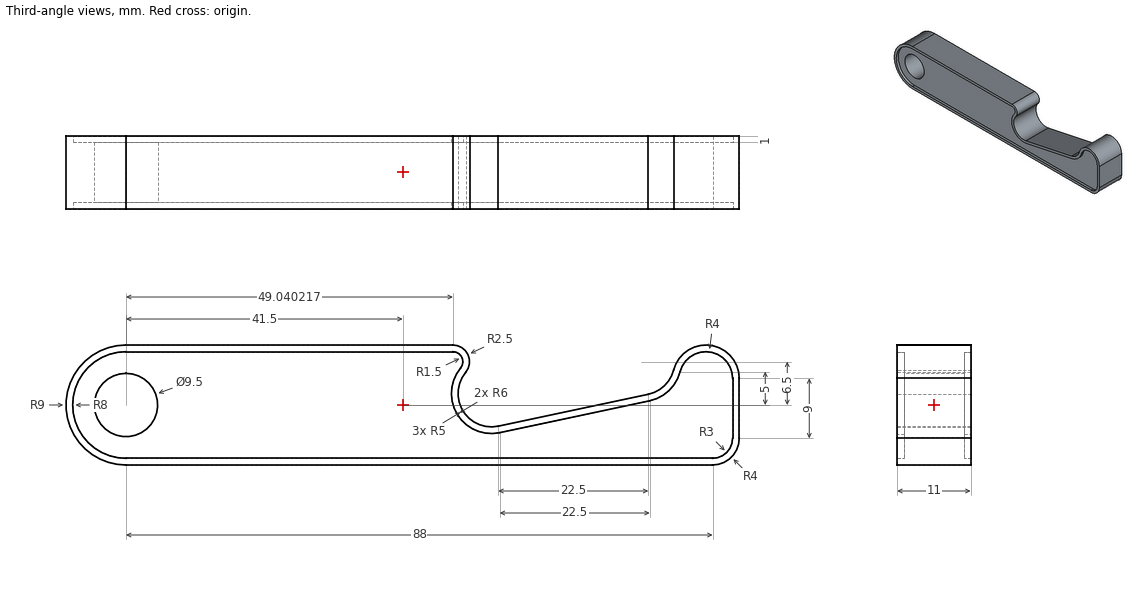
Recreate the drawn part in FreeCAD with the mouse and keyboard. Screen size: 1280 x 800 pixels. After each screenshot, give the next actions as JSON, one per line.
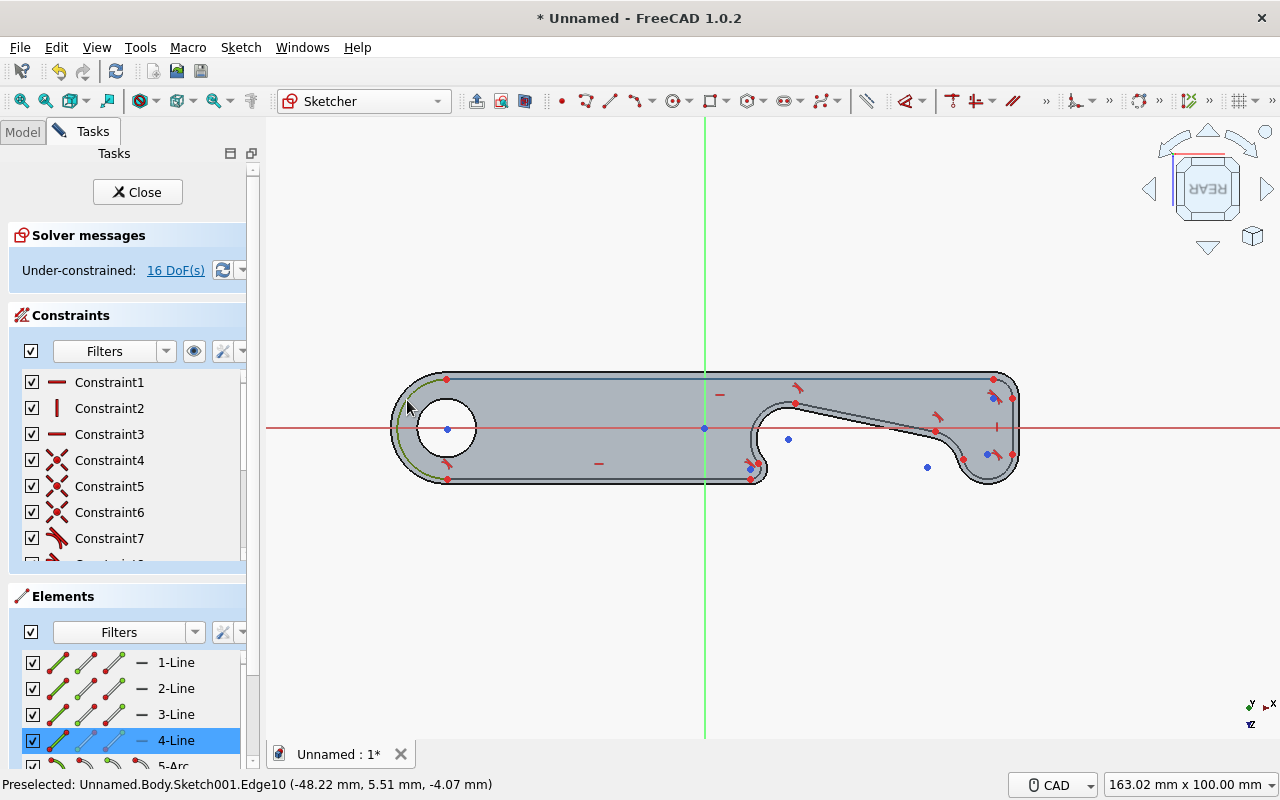
{"action": "key", "text": "t"}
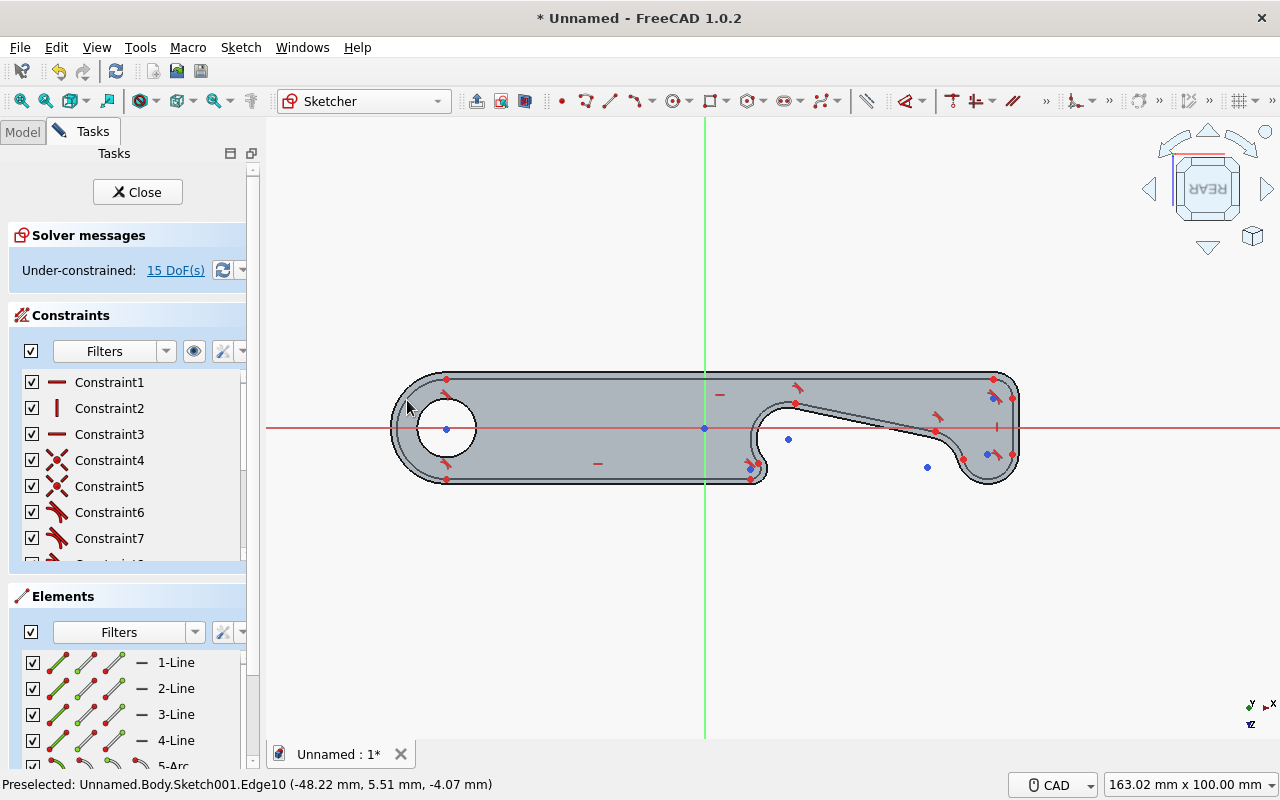
{"action": "scroll", "coordinate": [760, 474], "scroll_direction": "up", "scroll_amount": 2}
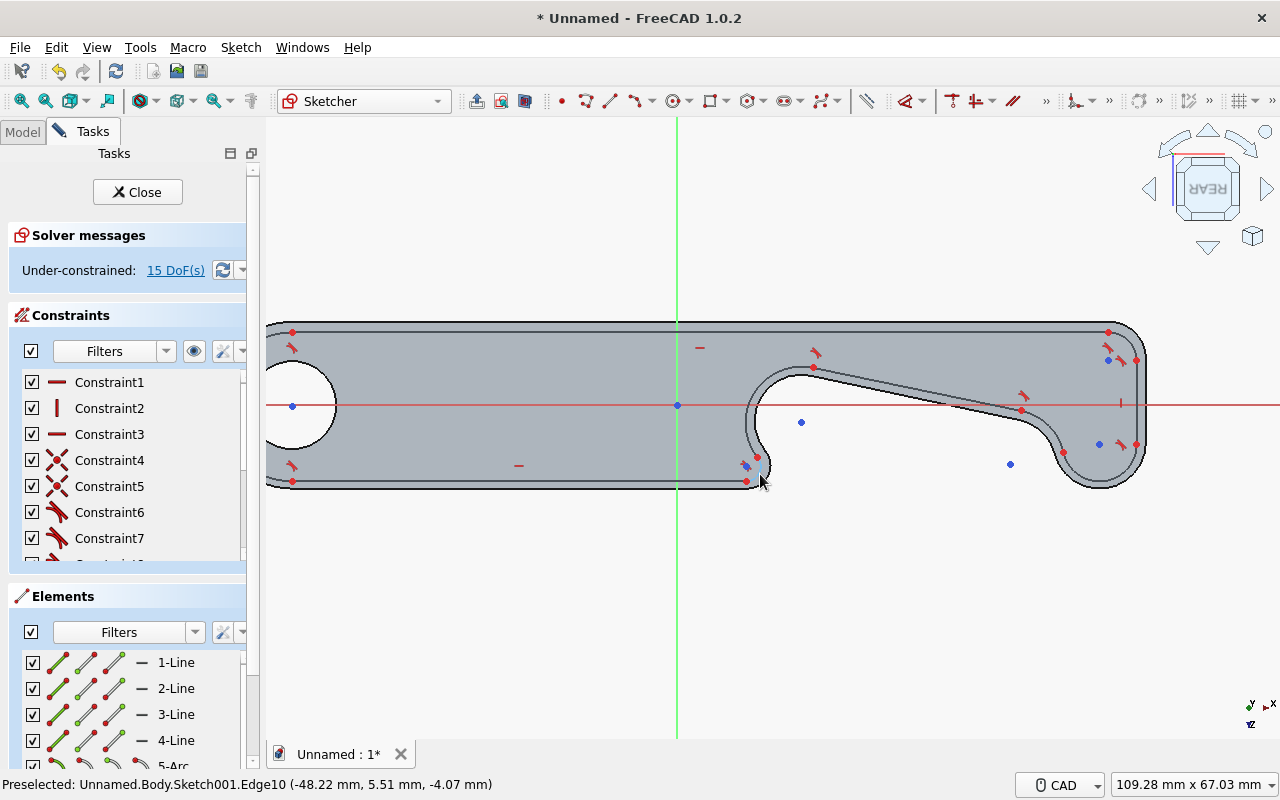
{"action": "left_click", "coordinate": [759, 473]}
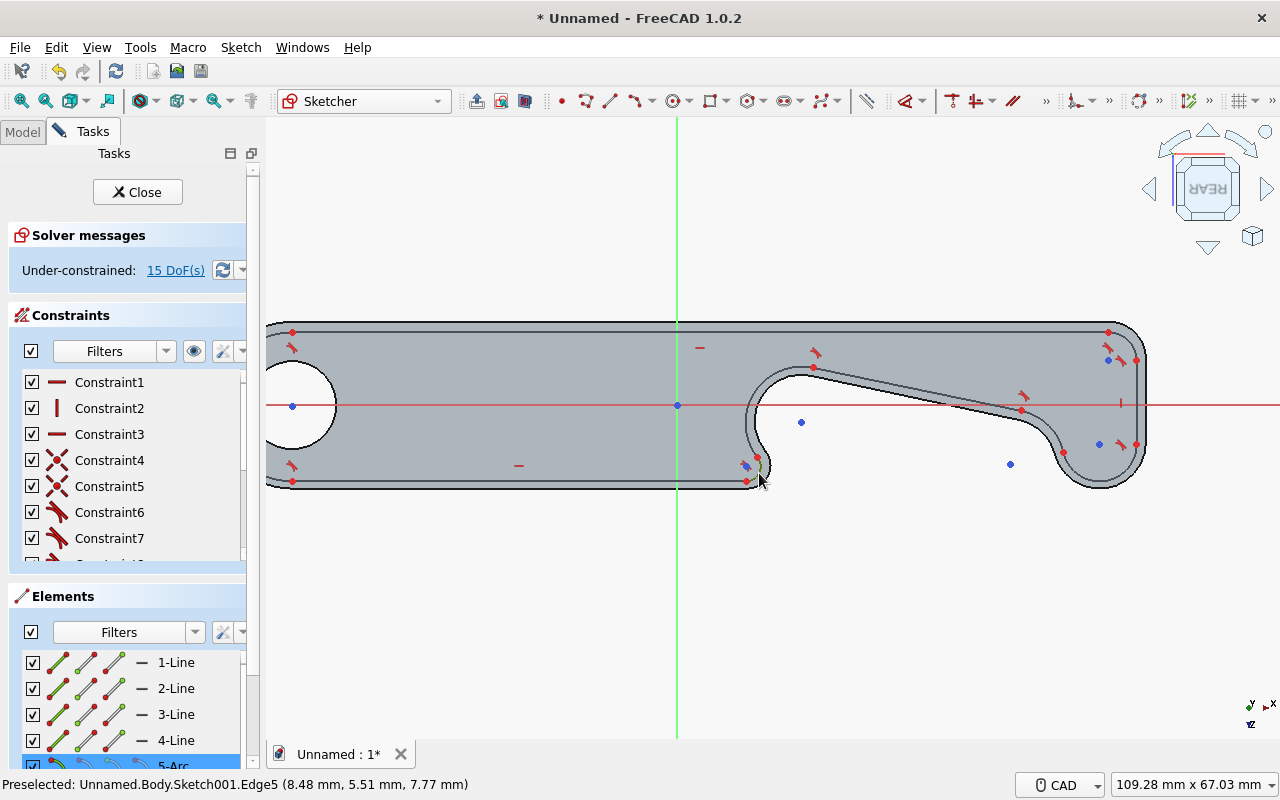
{"action": "left_click", "coordinate": [773, 374]}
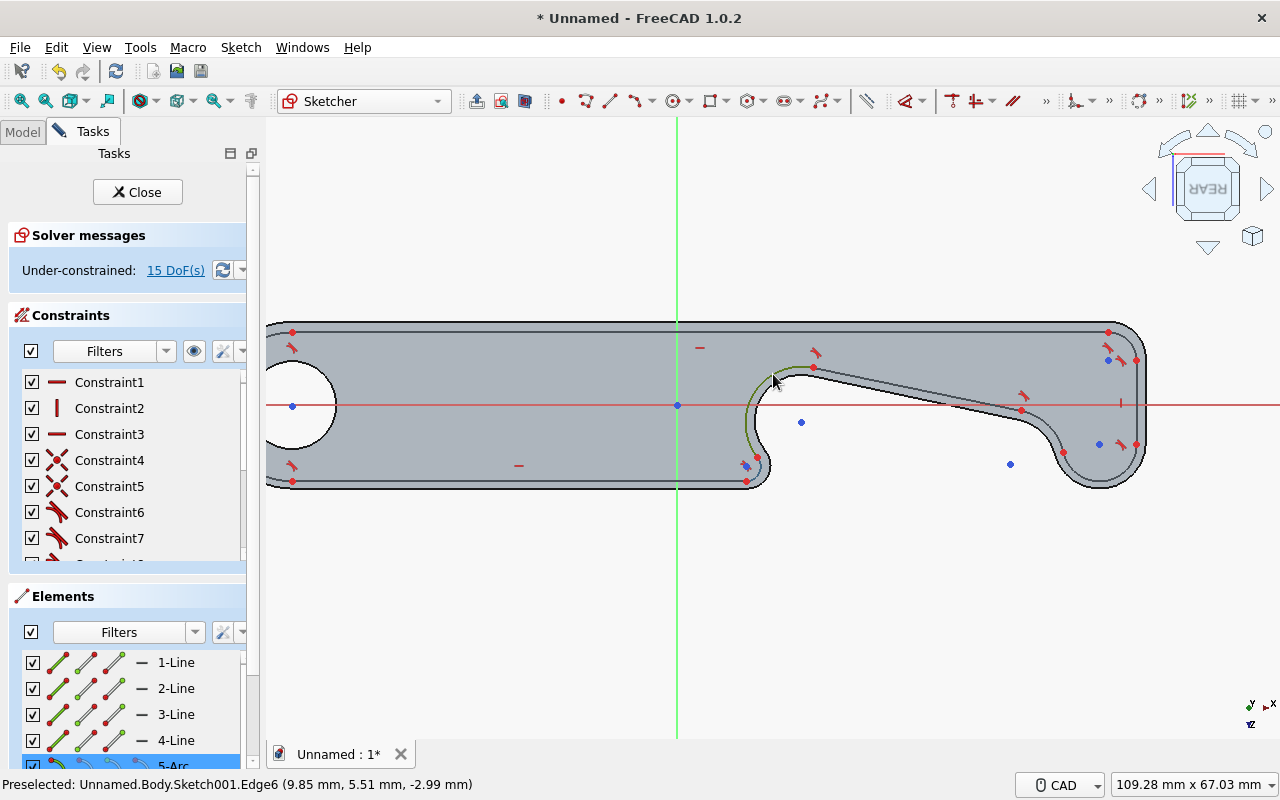
{"action": "key", "text": "t"}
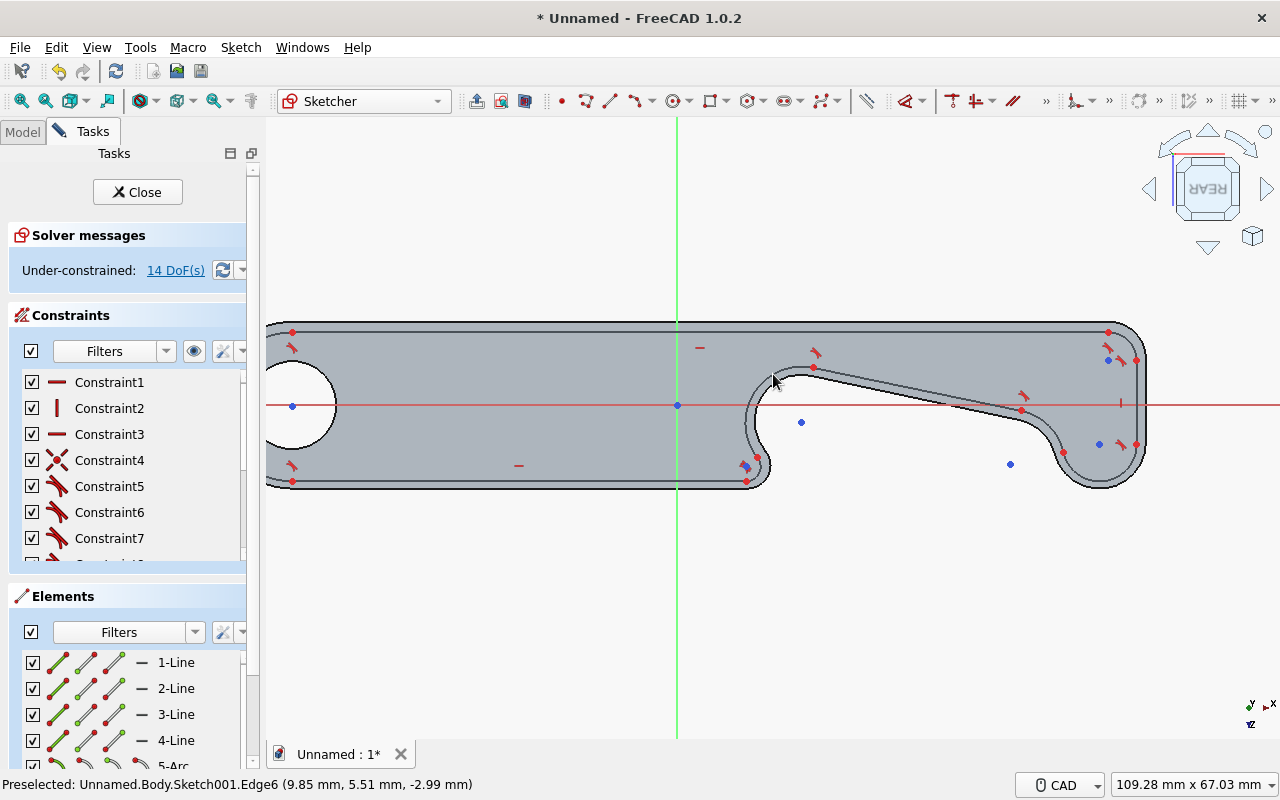
{"action": "left_click", "coordinate": [1057, 435]}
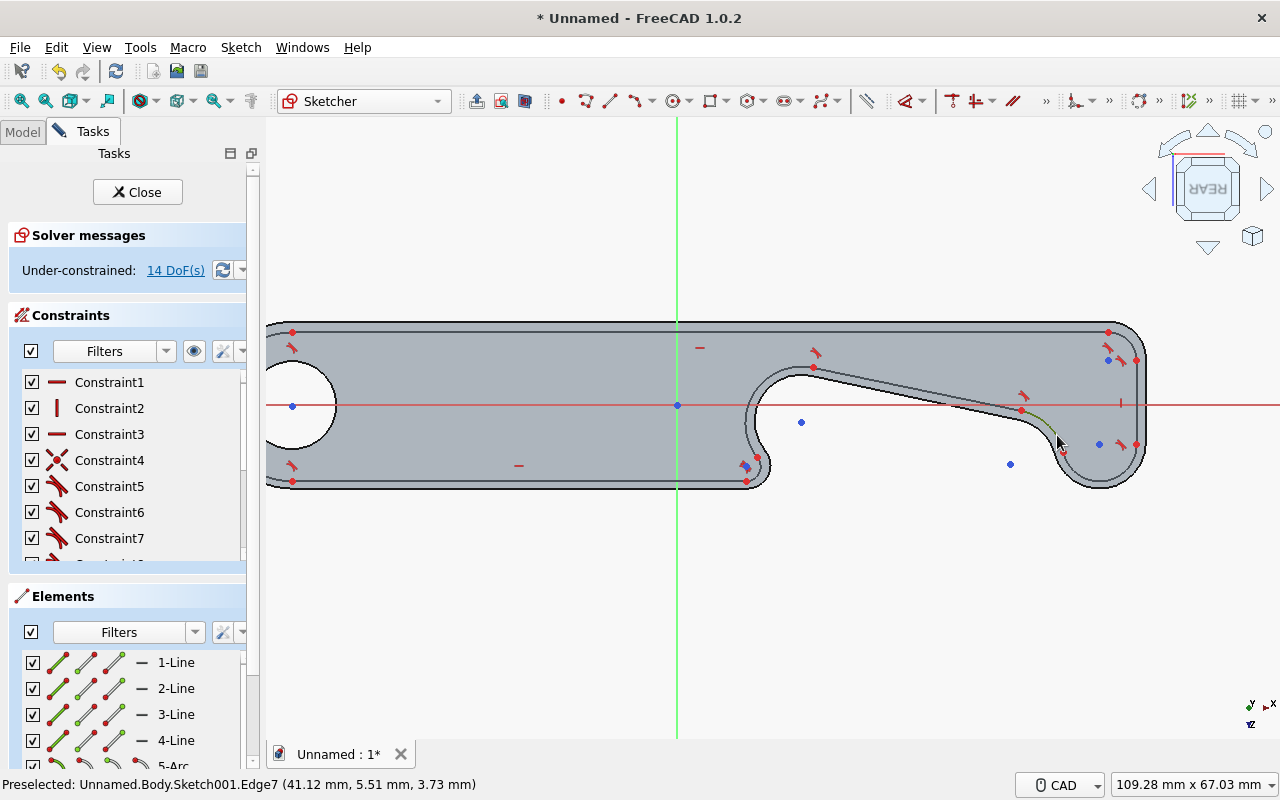
{"action": "left_click", "coordinate": [1083, 477]}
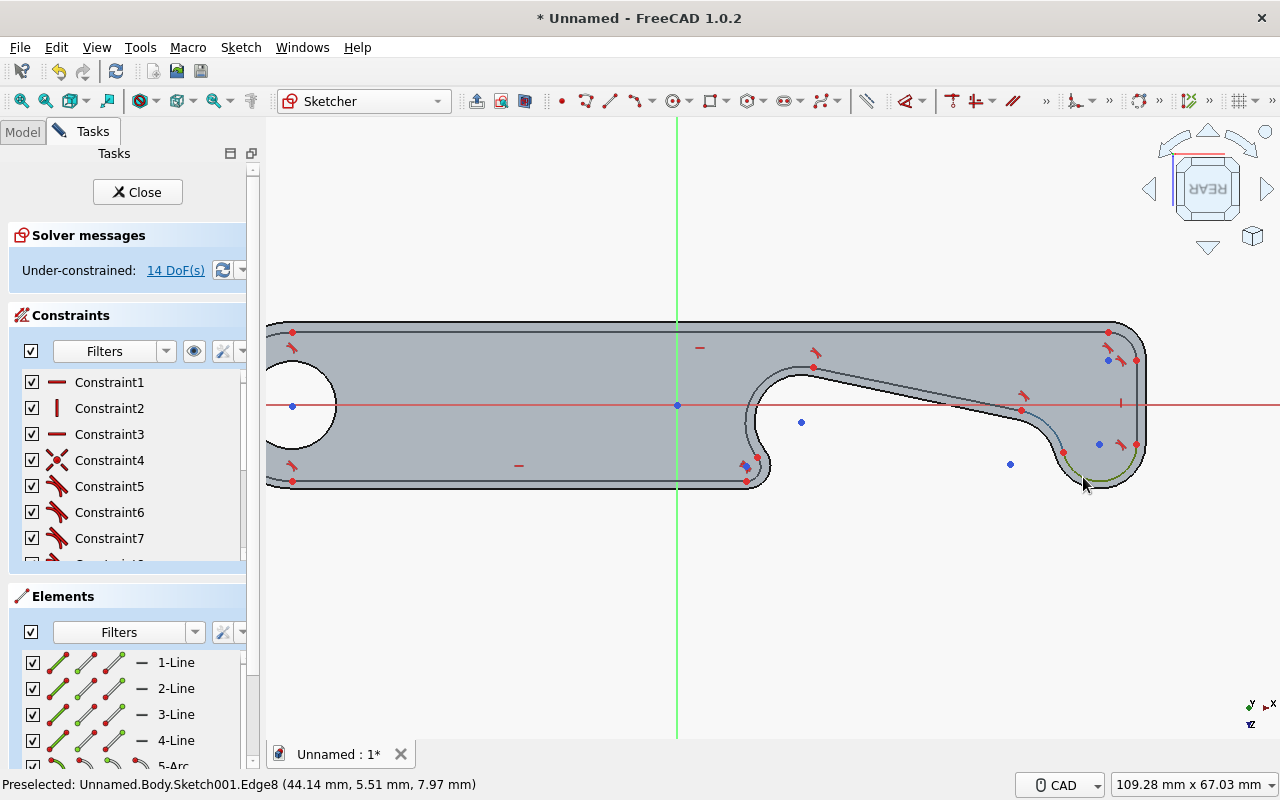
{"action": "key", "text": "t"}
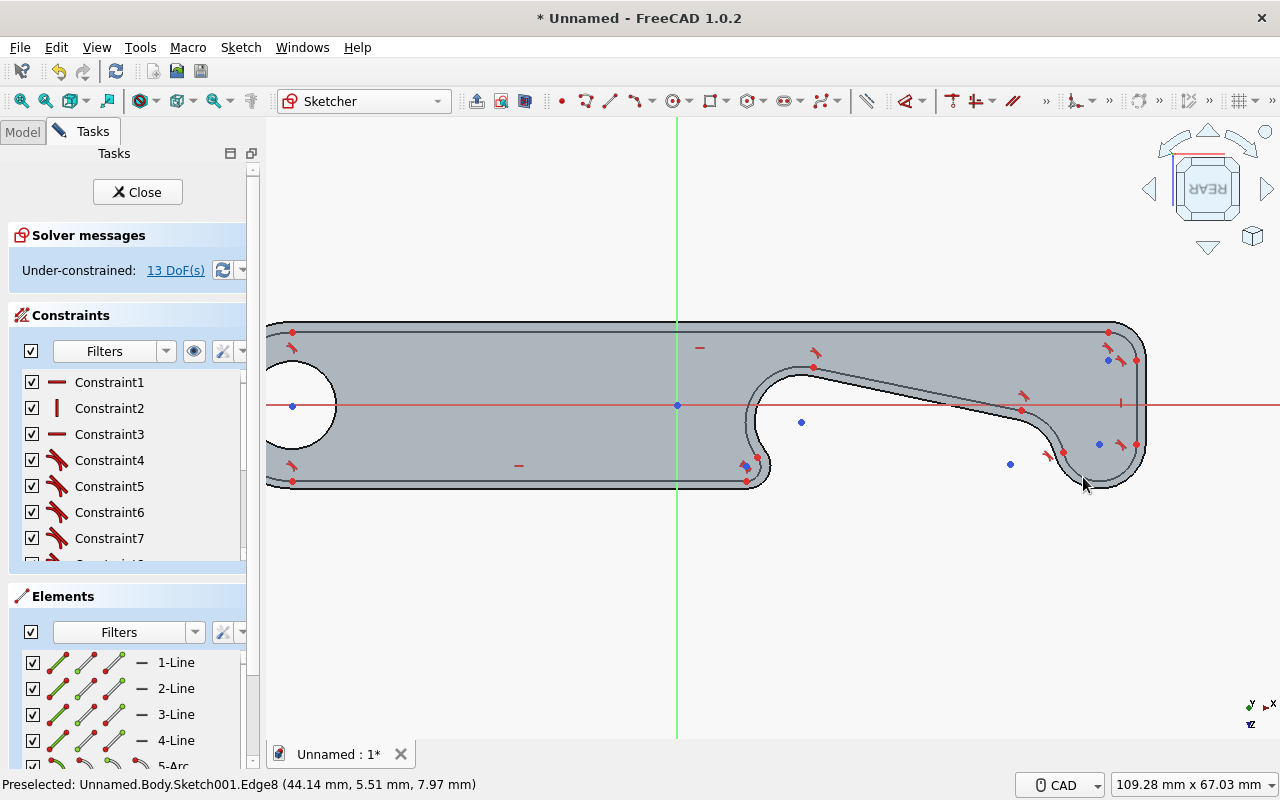
{"action": "left_click", "coordinate": [773, 374]}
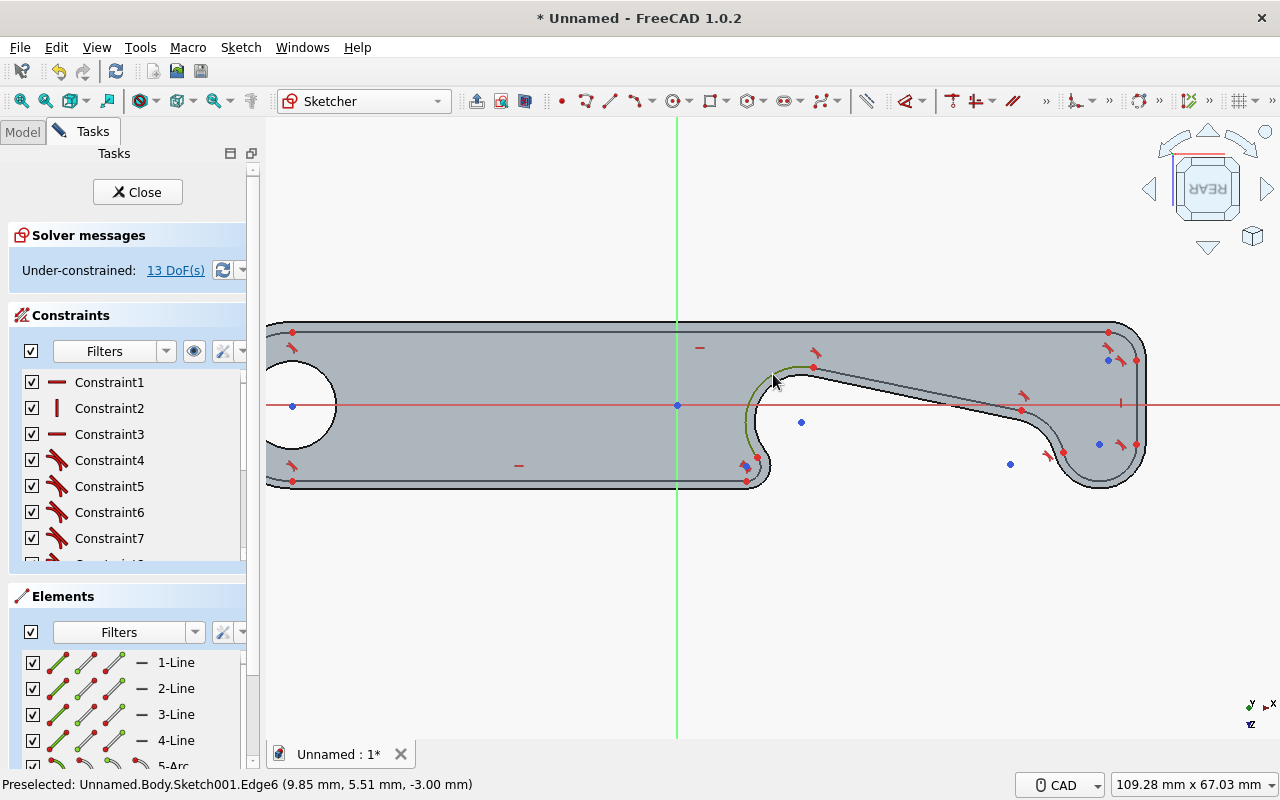
{"action": "left_click", "coordinate": [1056, 435]}